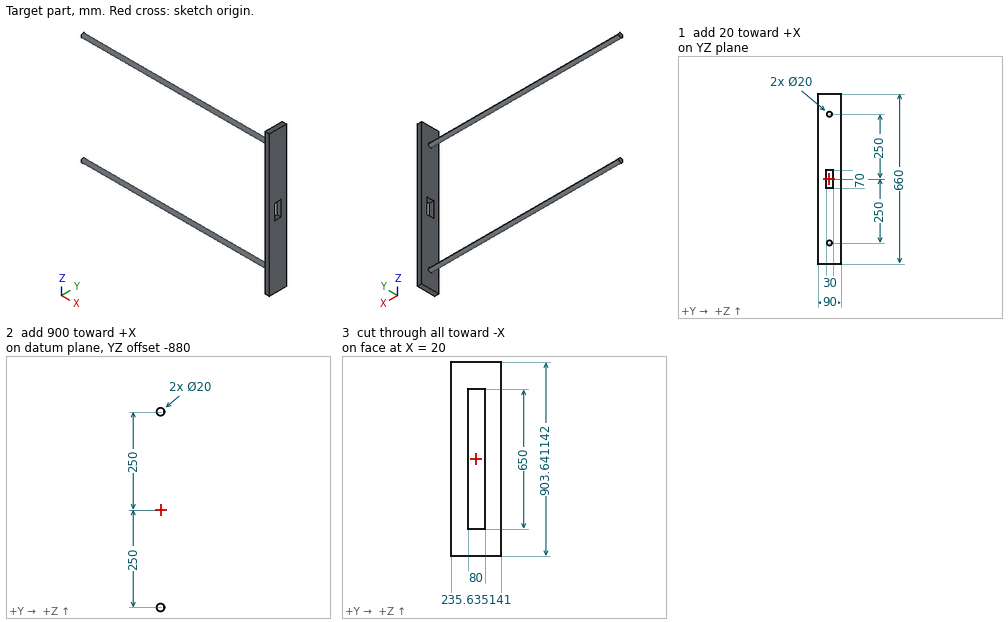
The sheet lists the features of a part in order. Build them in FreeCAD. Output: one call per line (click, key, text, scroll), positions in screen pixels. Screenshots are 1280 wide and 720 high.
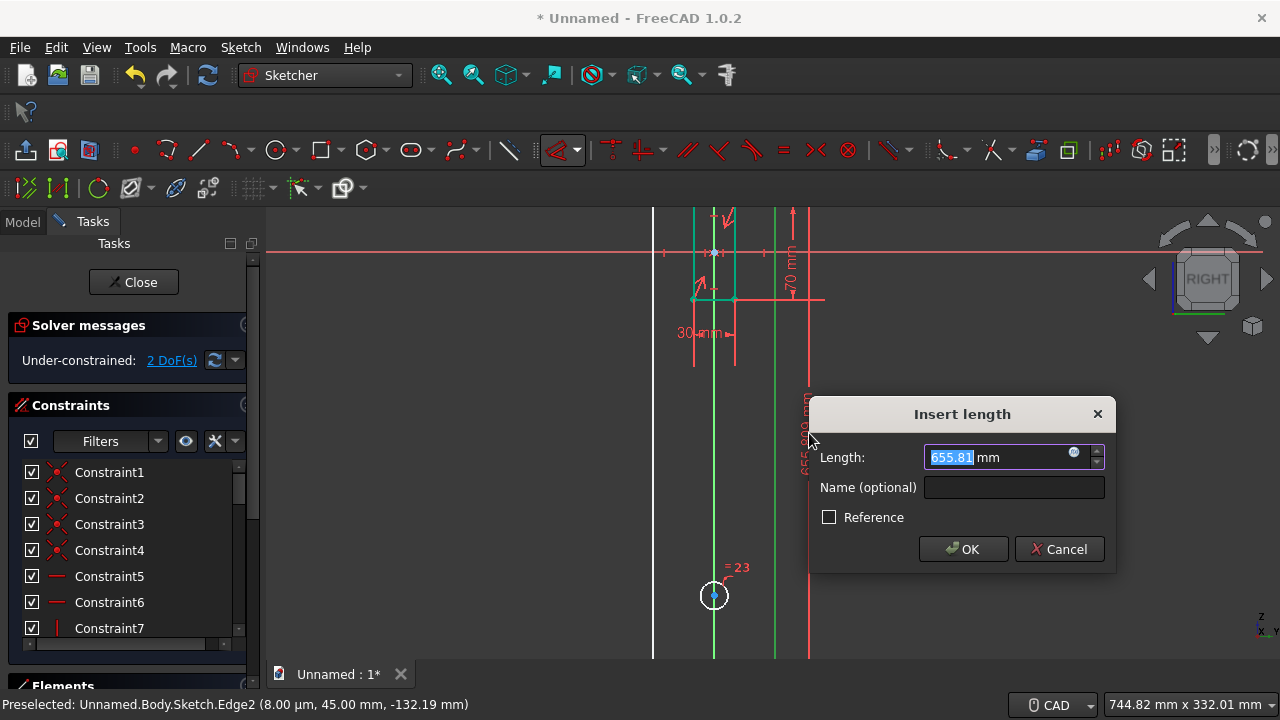
text(660)
key(Return)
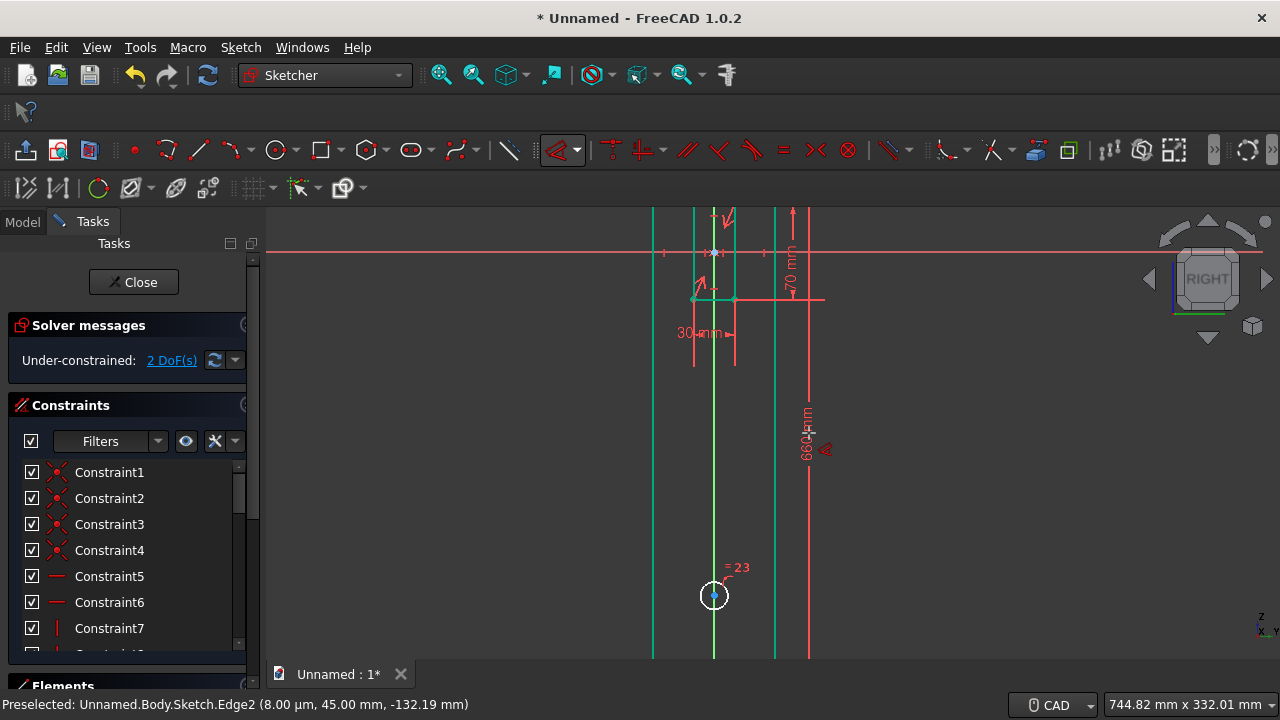
scroll(700, 511, down, 6)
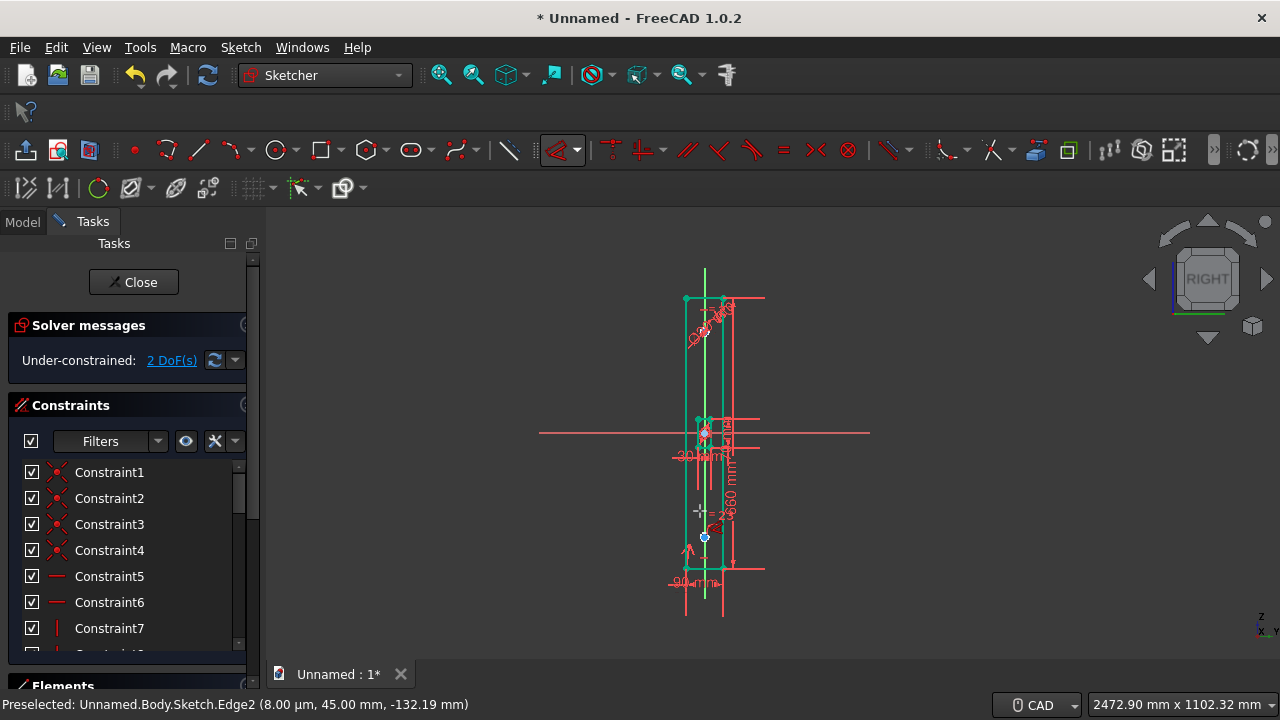
click(705, 332)
click(739, 383)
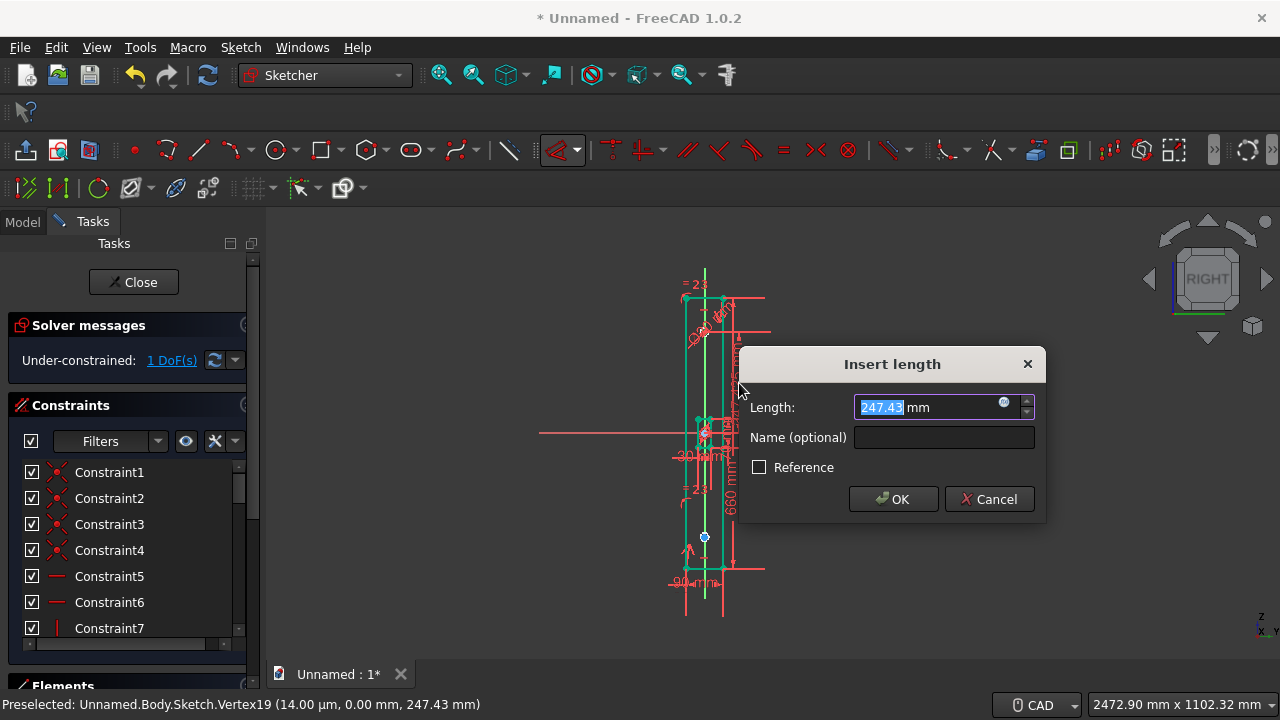
text(250)
key(Return)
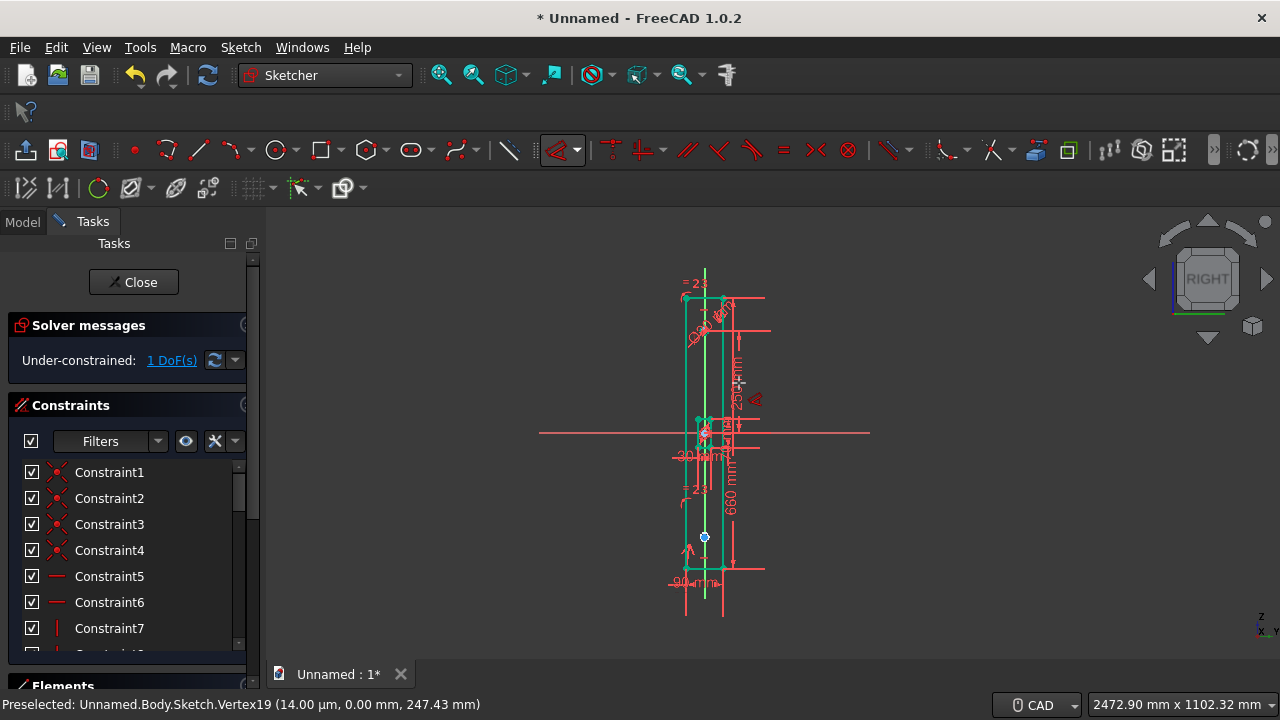
click(705, 537)
click(739, 509)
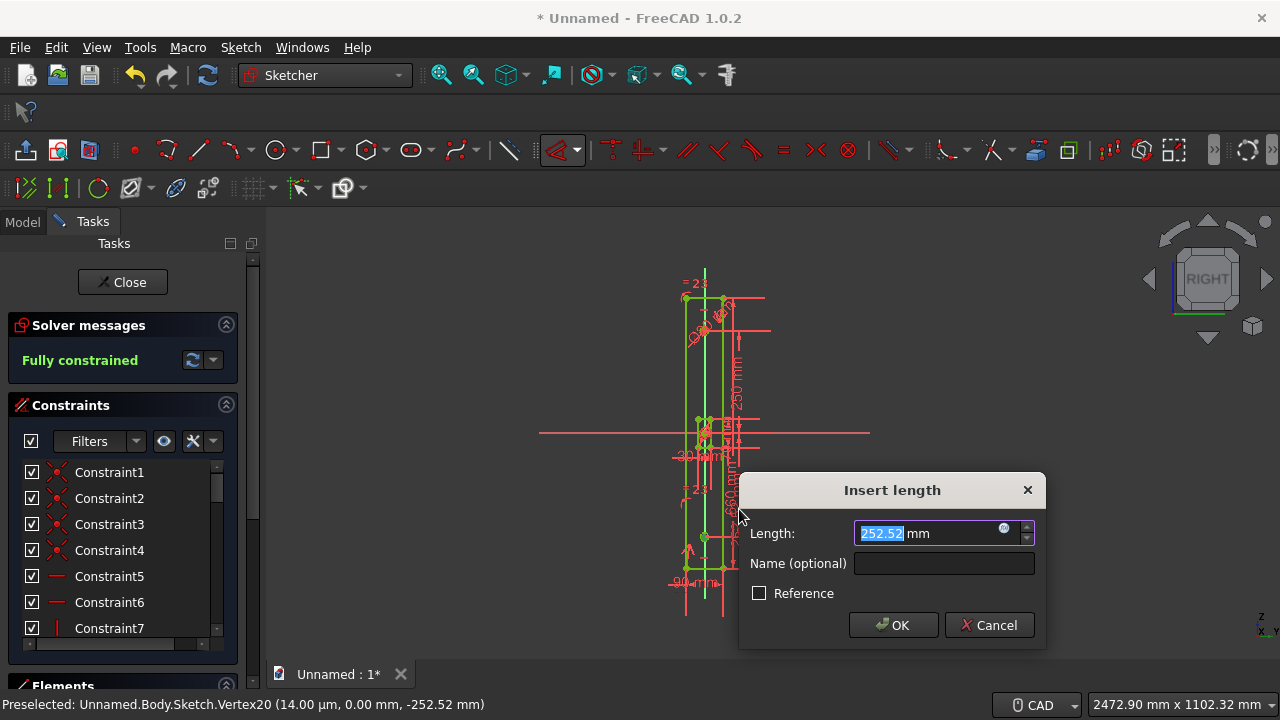
text(250)
key(Return)
key(Escape)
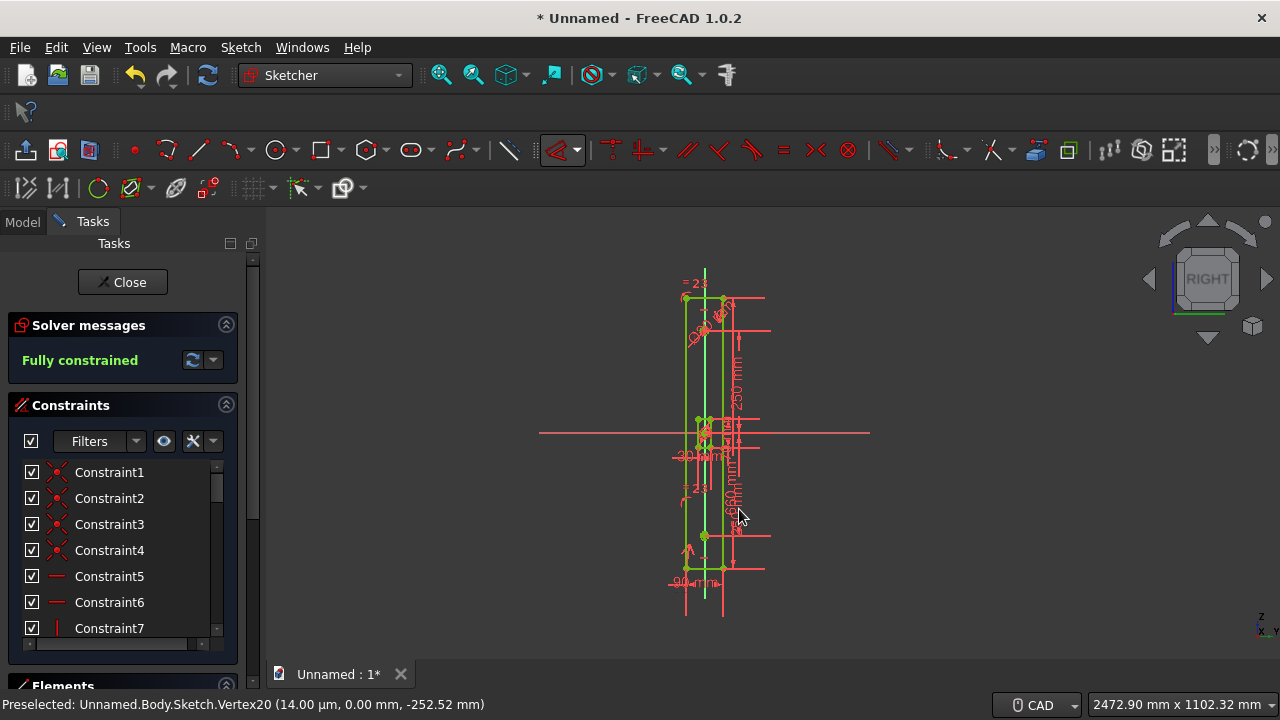
click(123, 282)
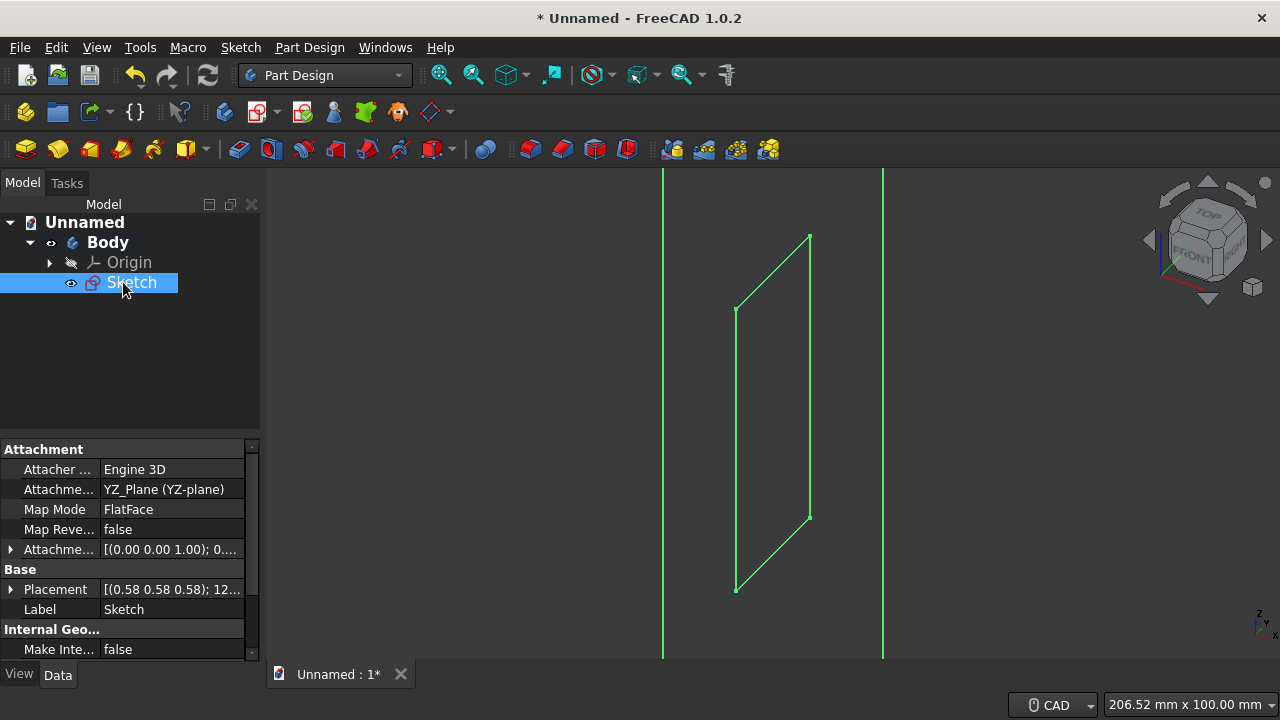
click(26, 150)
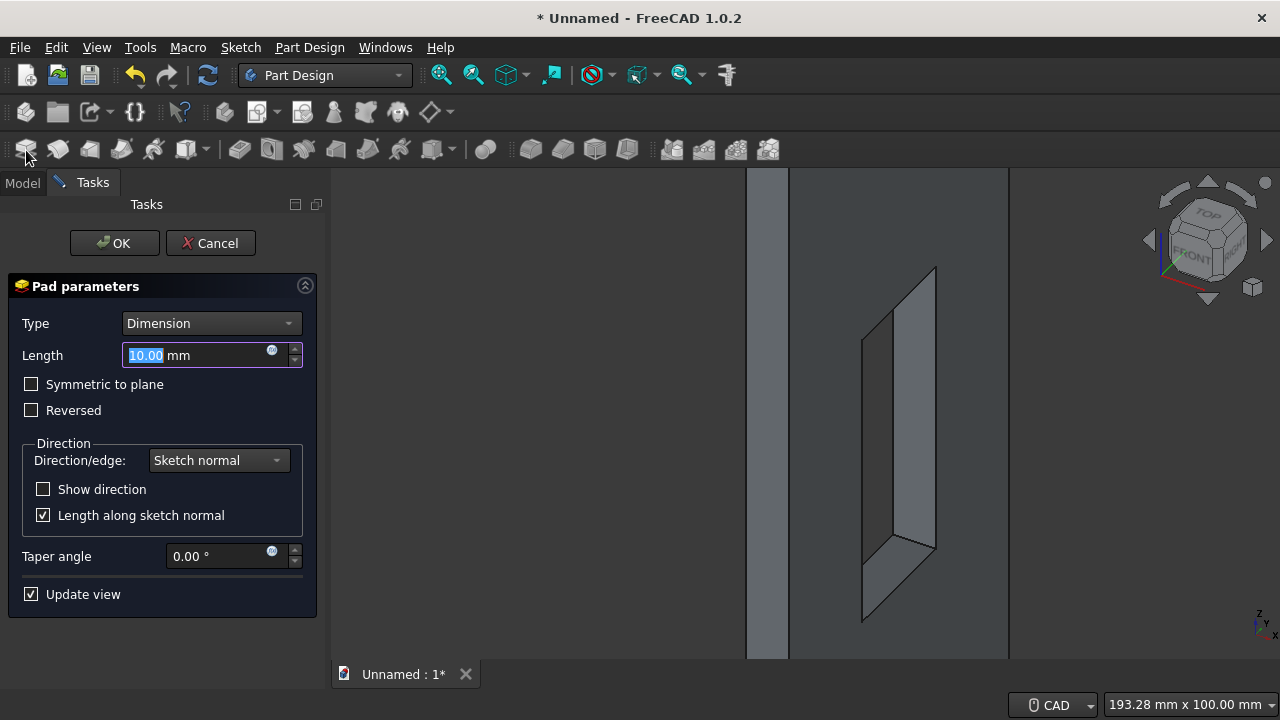
text(20)
key(Tab)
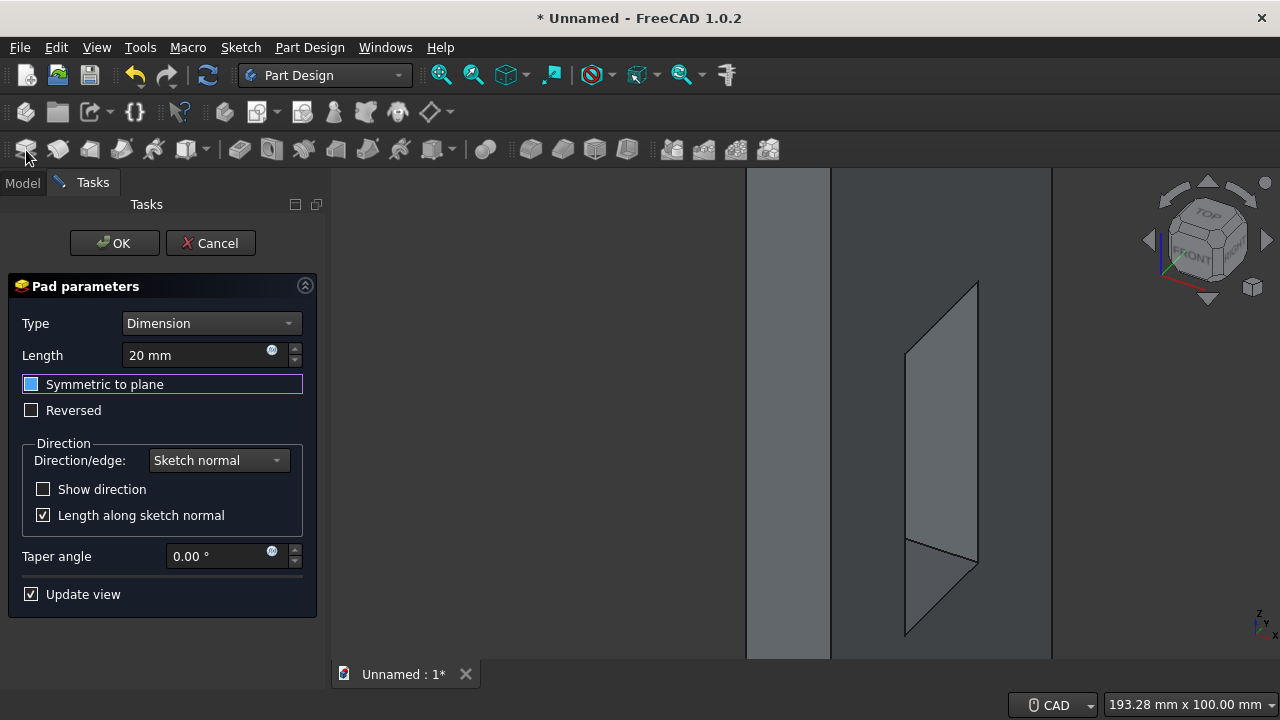
click(115, 243)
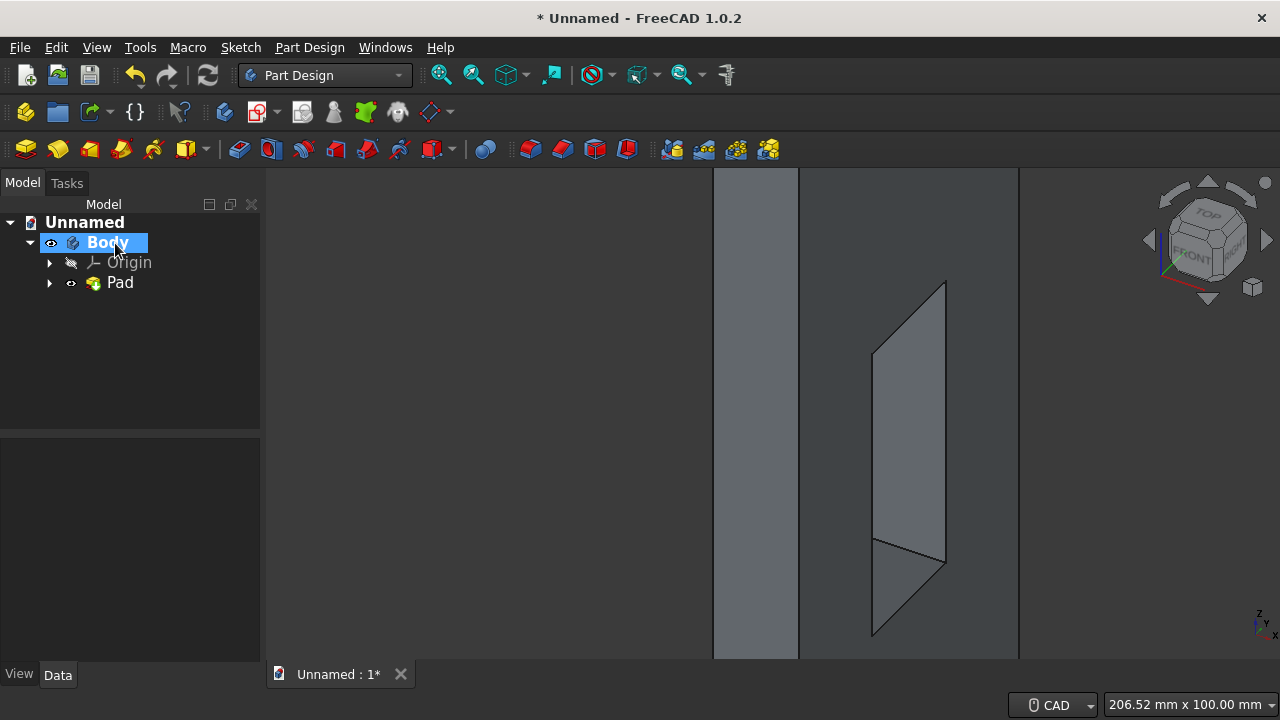
click(442, 76)